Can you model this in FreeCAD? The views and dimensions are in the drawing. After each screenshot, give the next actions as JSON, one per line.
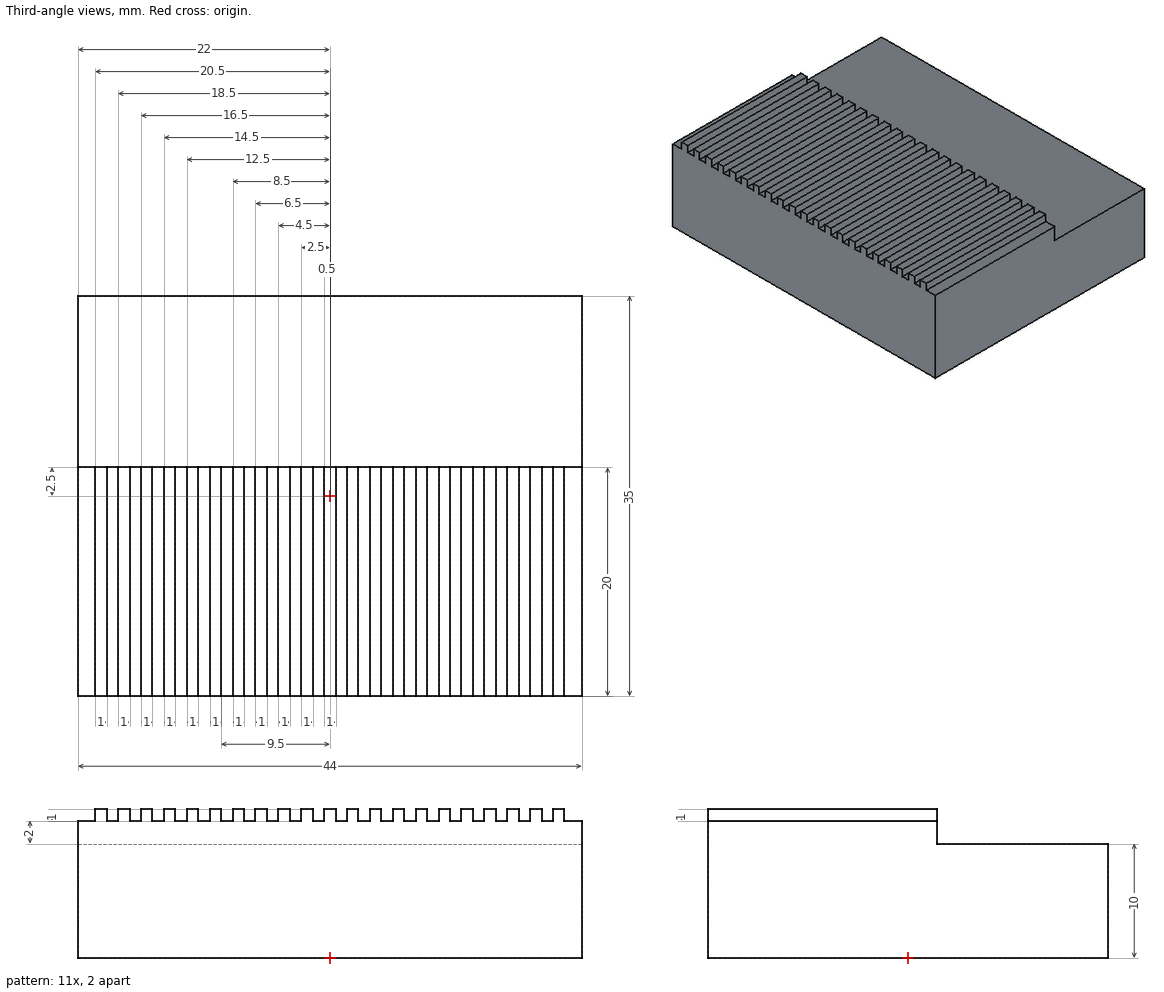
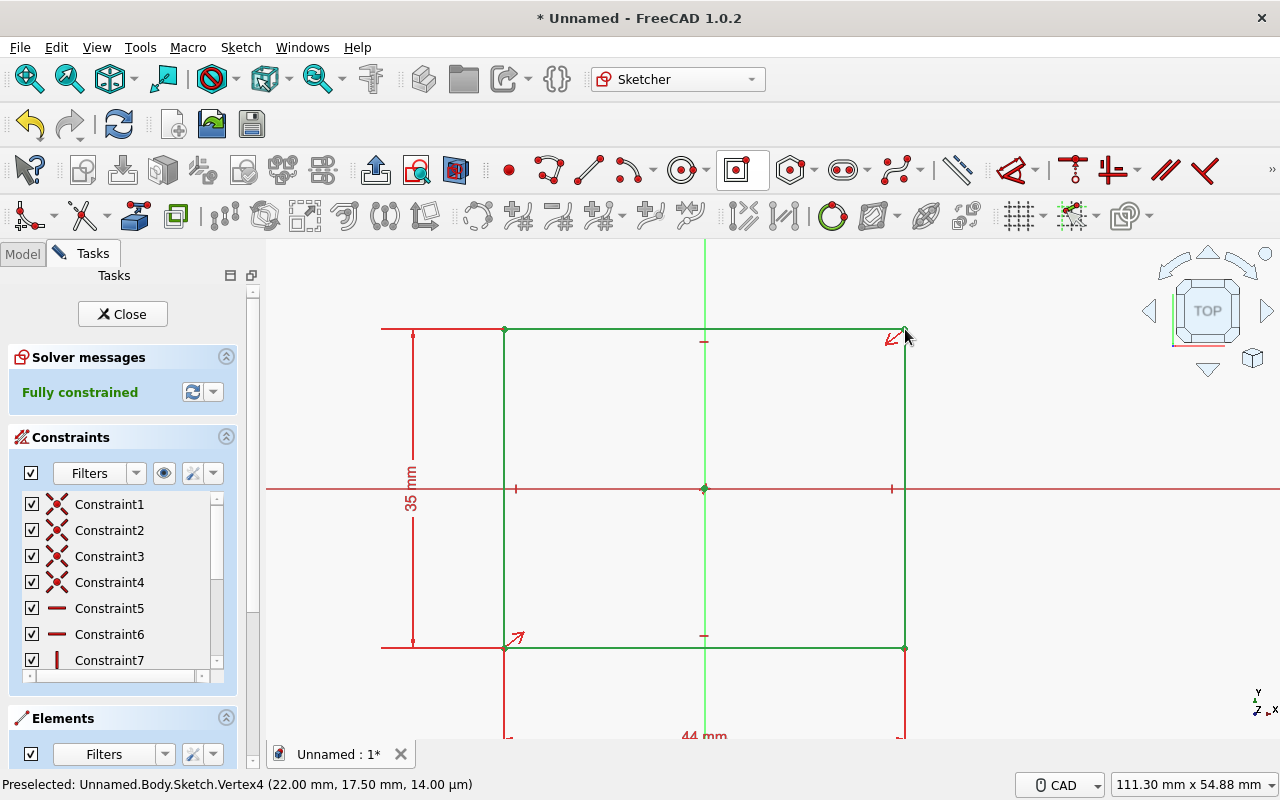
{"action": "left_click", "coordinate": [123, 314]}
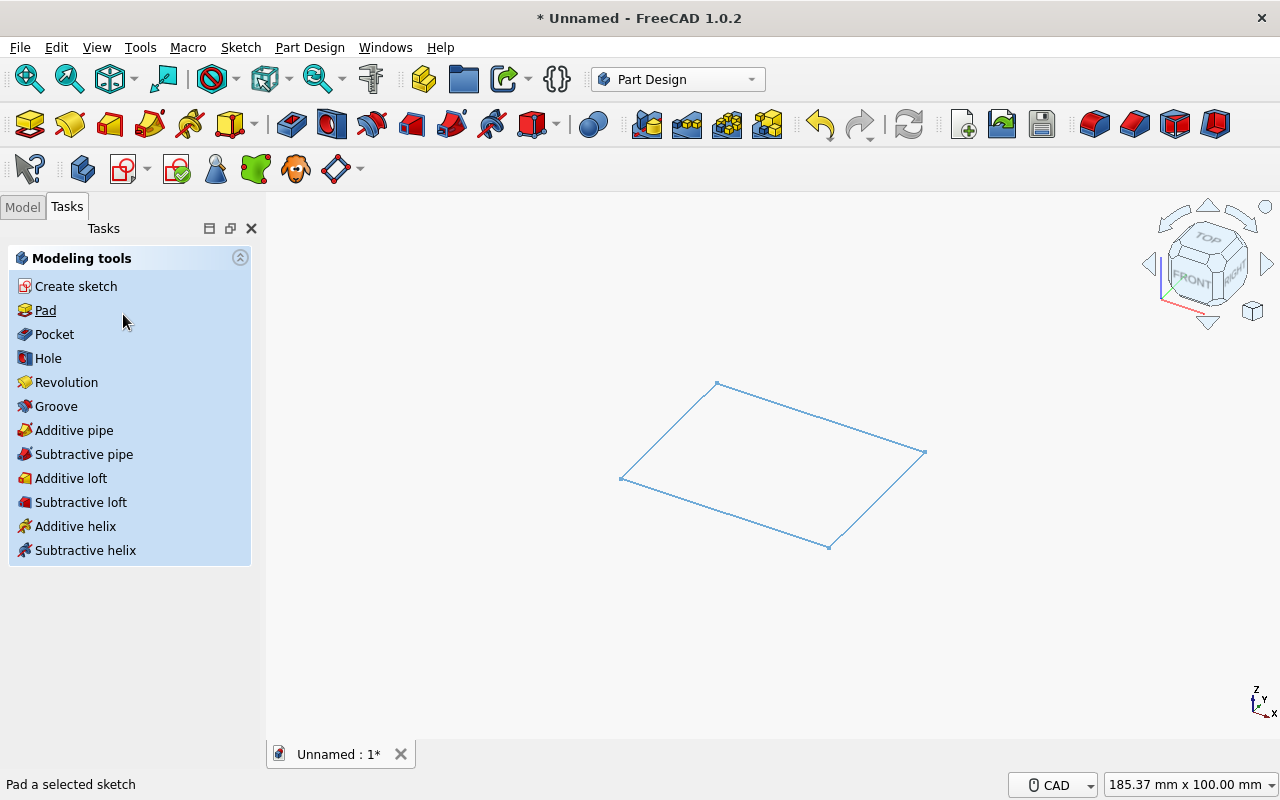
{"action": "left_click", "coordinate": [30, 124]}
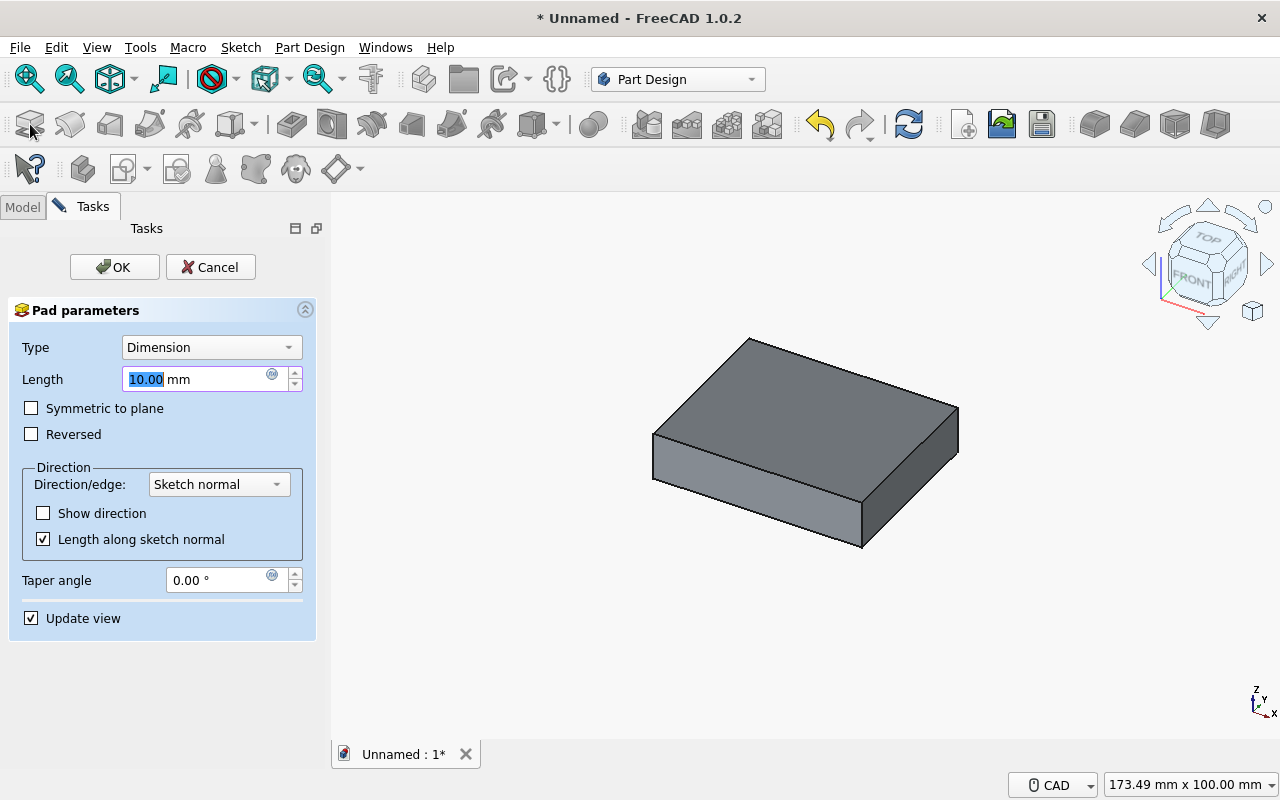
{"action": "type", "text": "10"}
{"action": "key", "text": "Tab"}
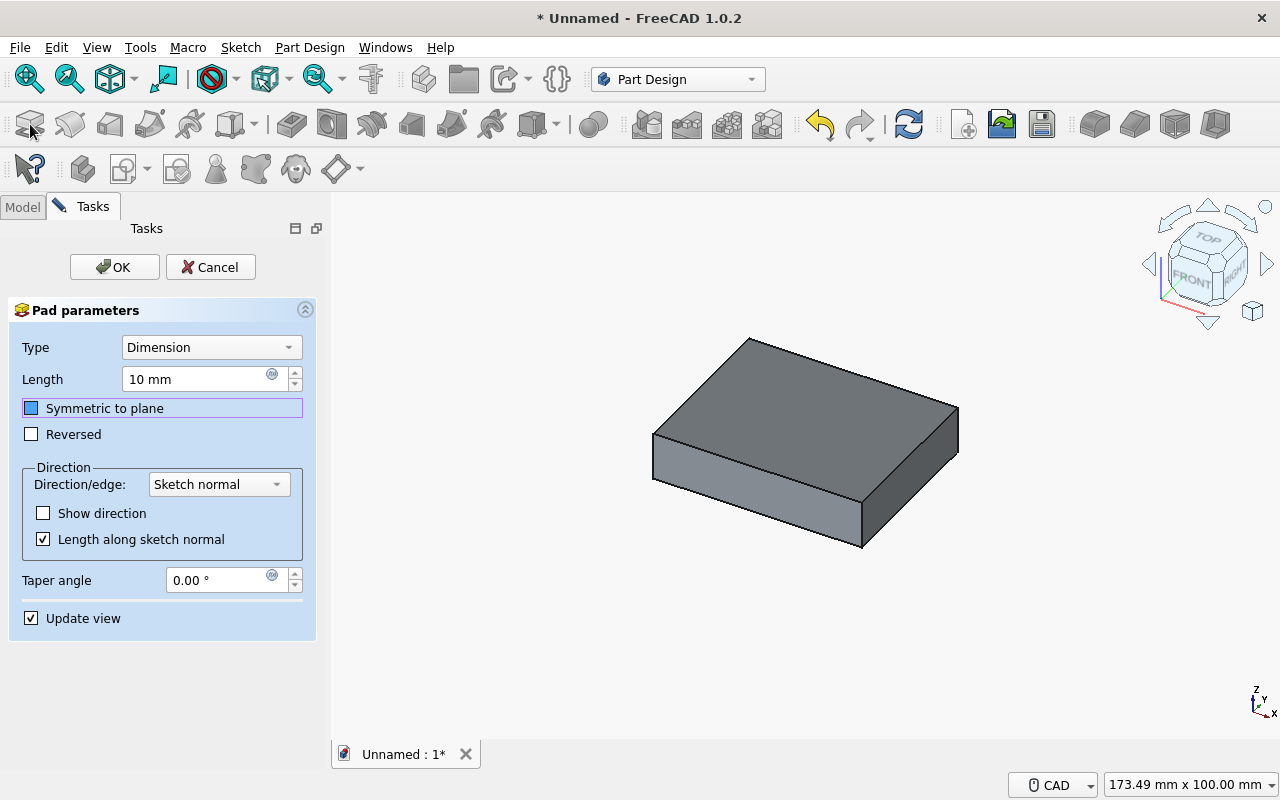
{"action": "left_click", "coordinate": [115, 267]}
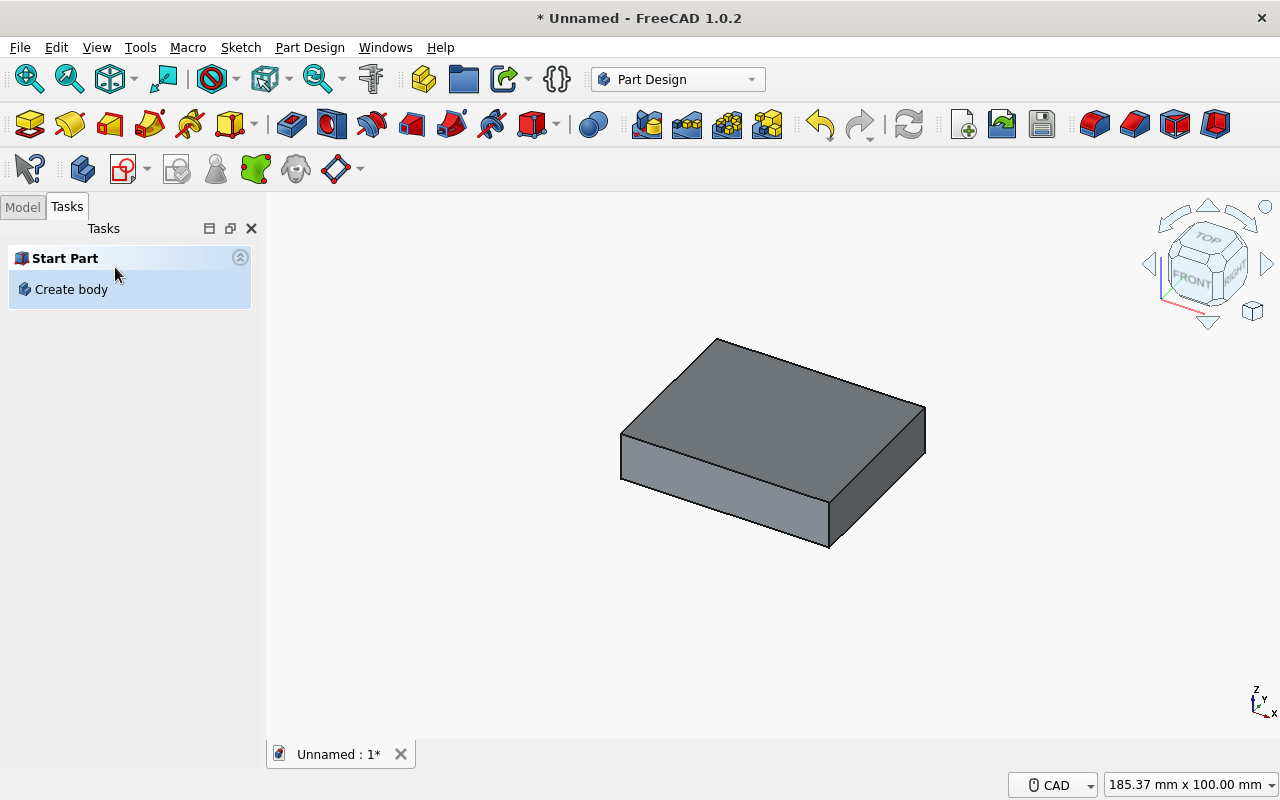
{"action": "left_click", "coordinate": [30, 80]}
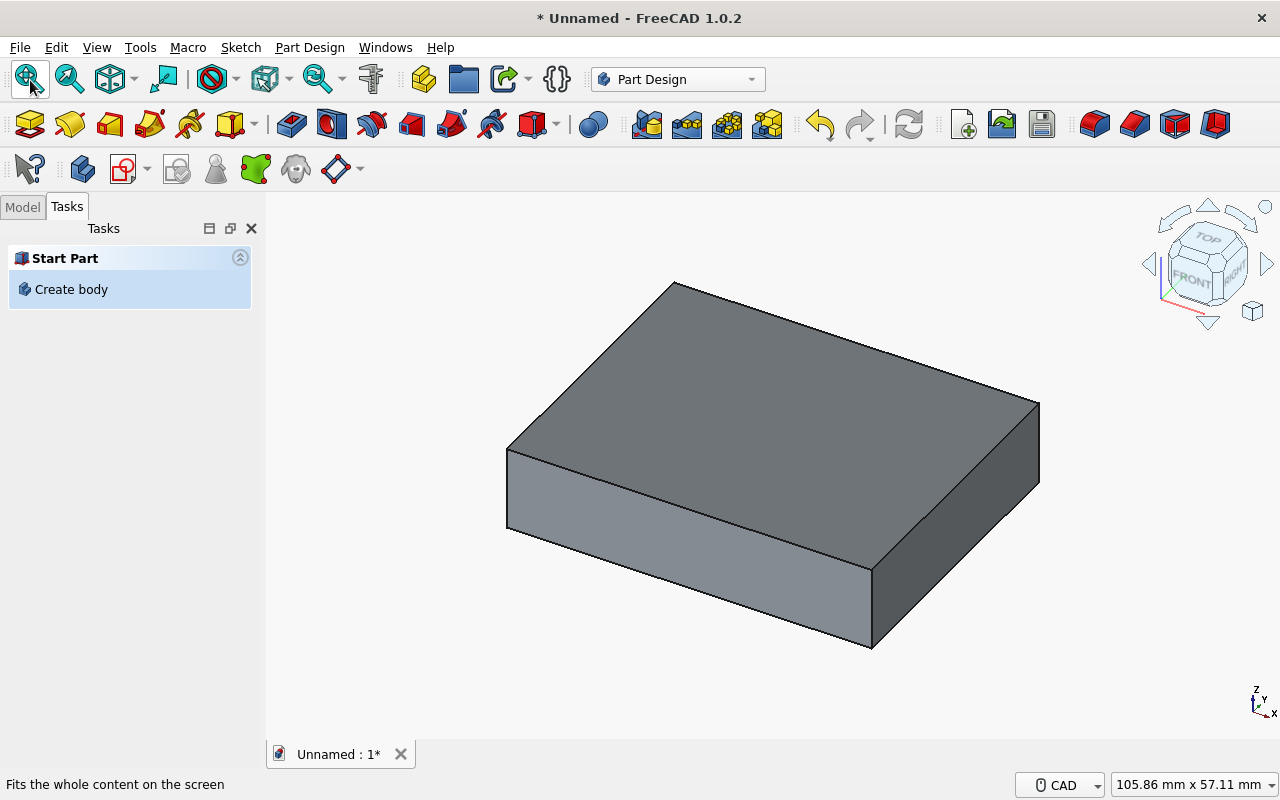
{"action": "left_click", "coordinate": [773, 425]}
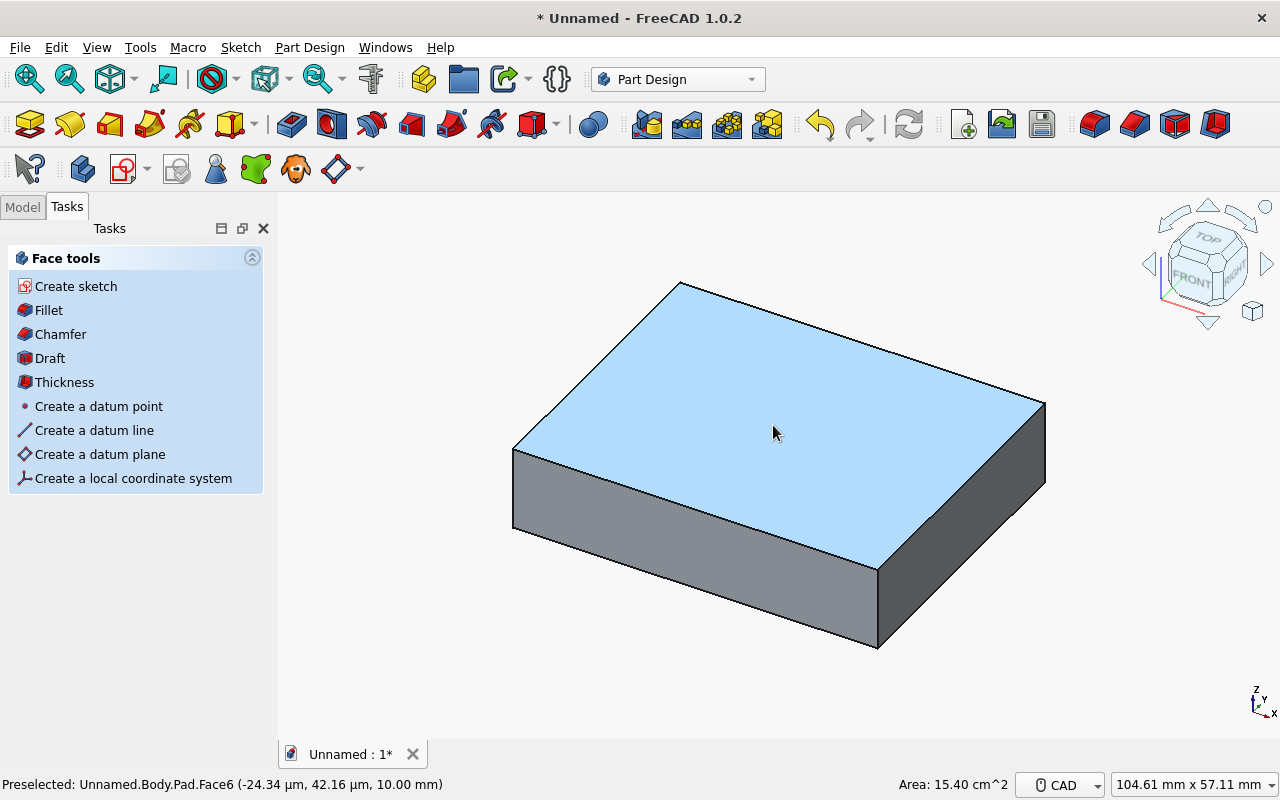
{"action": "left_click", "coordinate": [124, 170]}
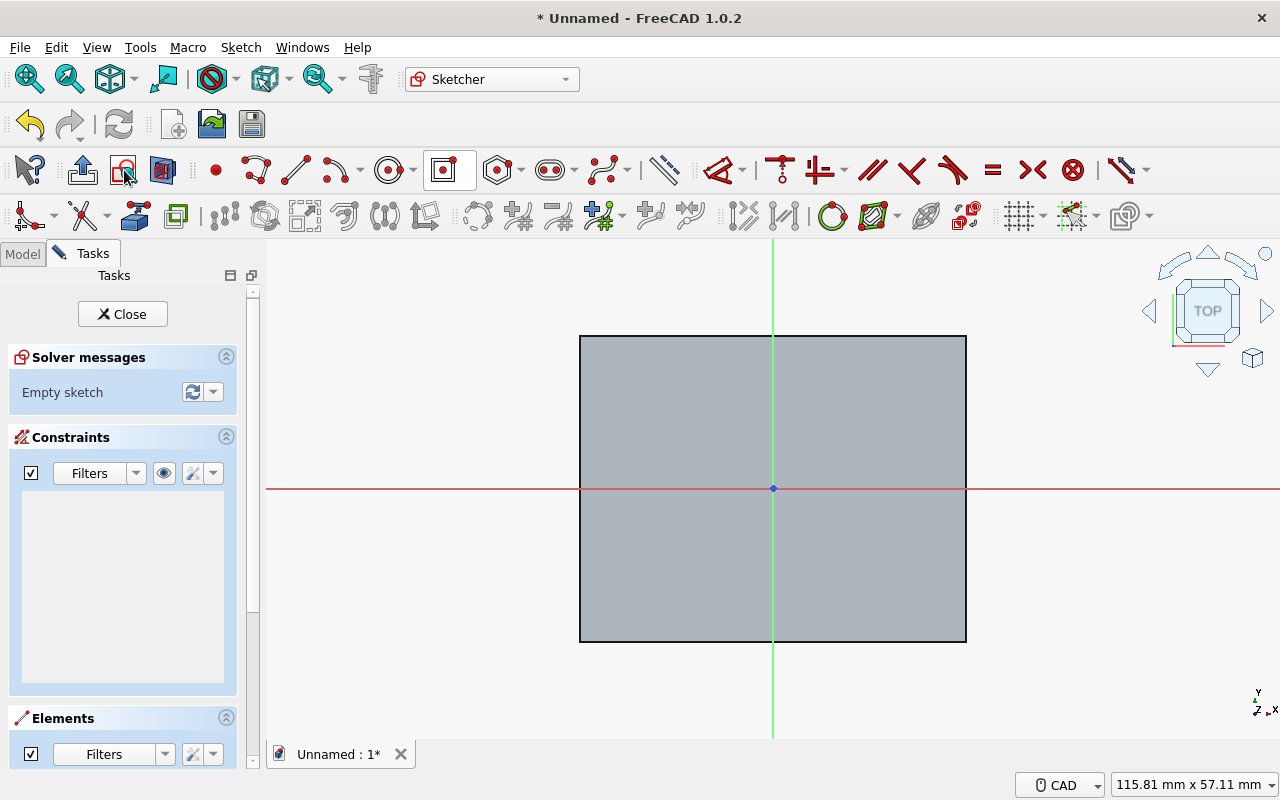
{"action": "scroll", "coordinate": [912, 688], "scroll_direction": "up", "scroll_amount": 2}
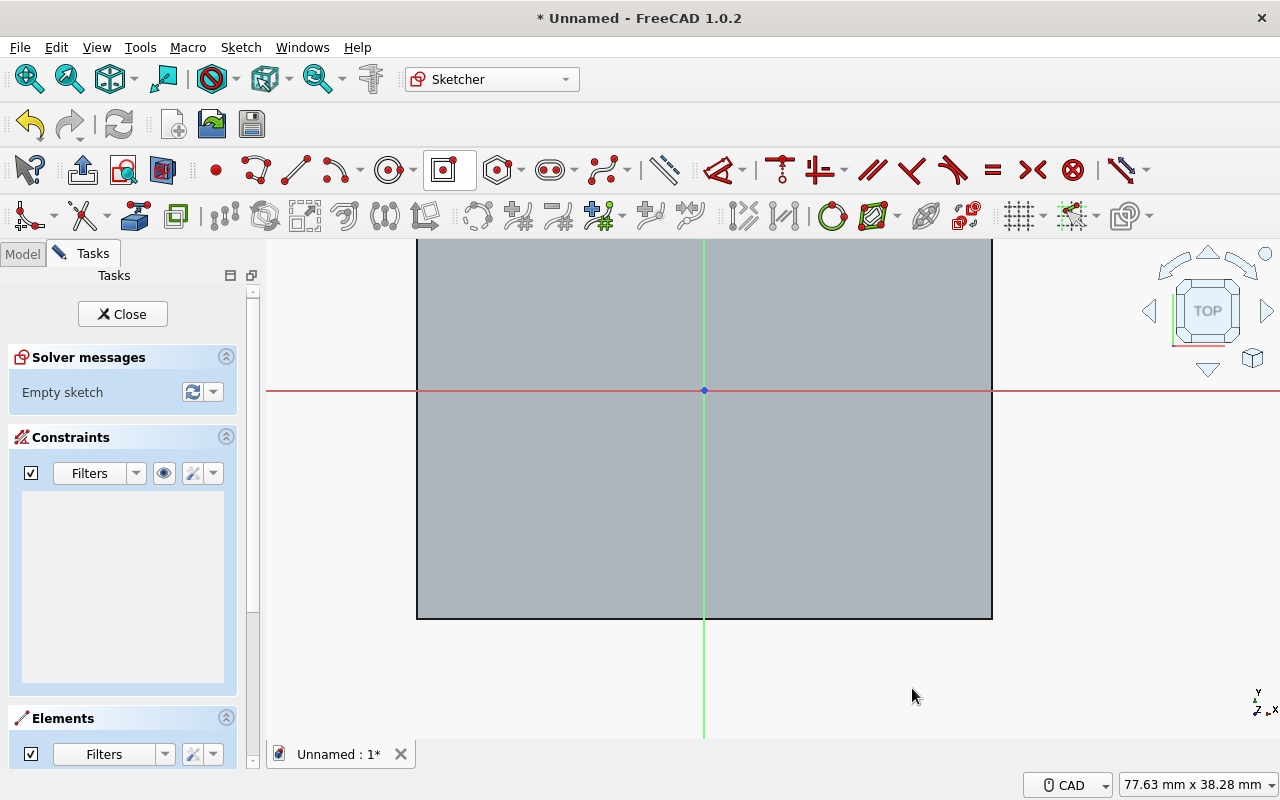
{"action": "key", "text": "g r"}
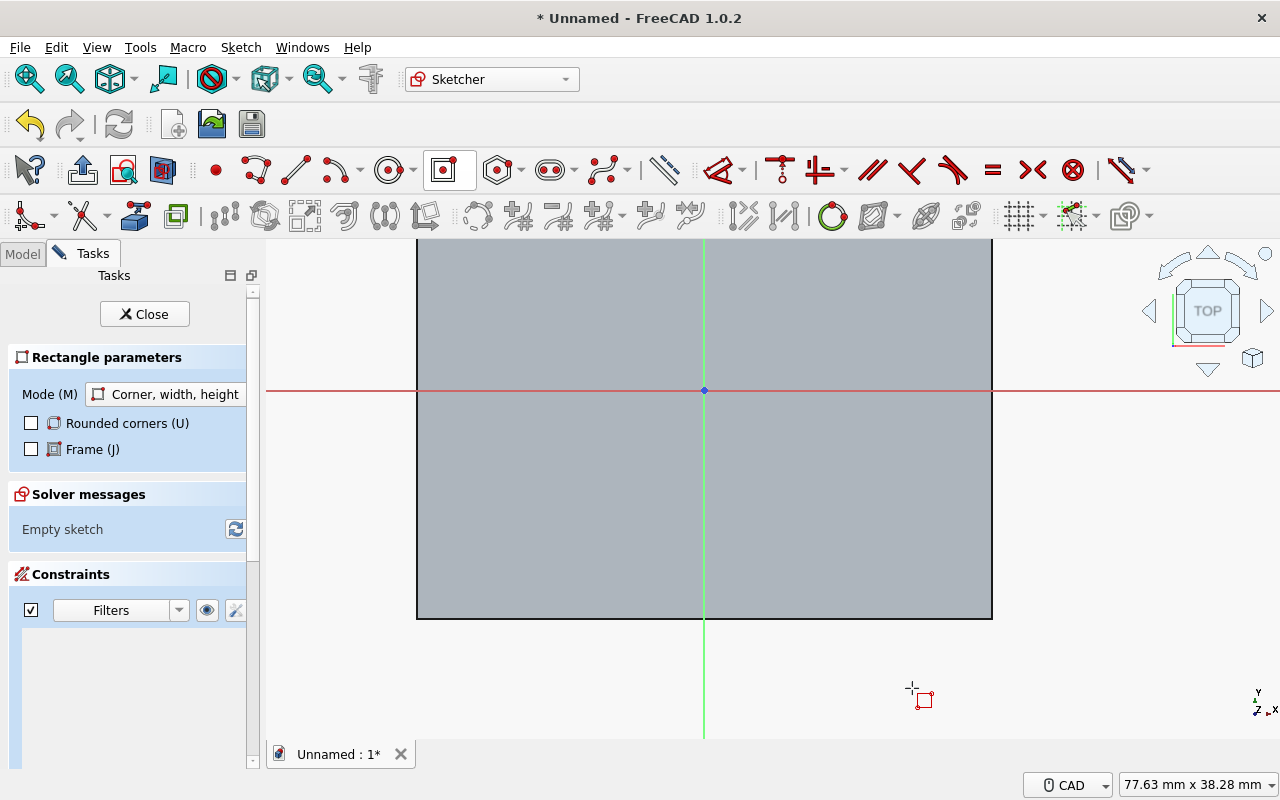
{"action": "left_click", "coordinate": [417, 358]}
{"action": "mouse_move", "coordinate": [992, 619]}